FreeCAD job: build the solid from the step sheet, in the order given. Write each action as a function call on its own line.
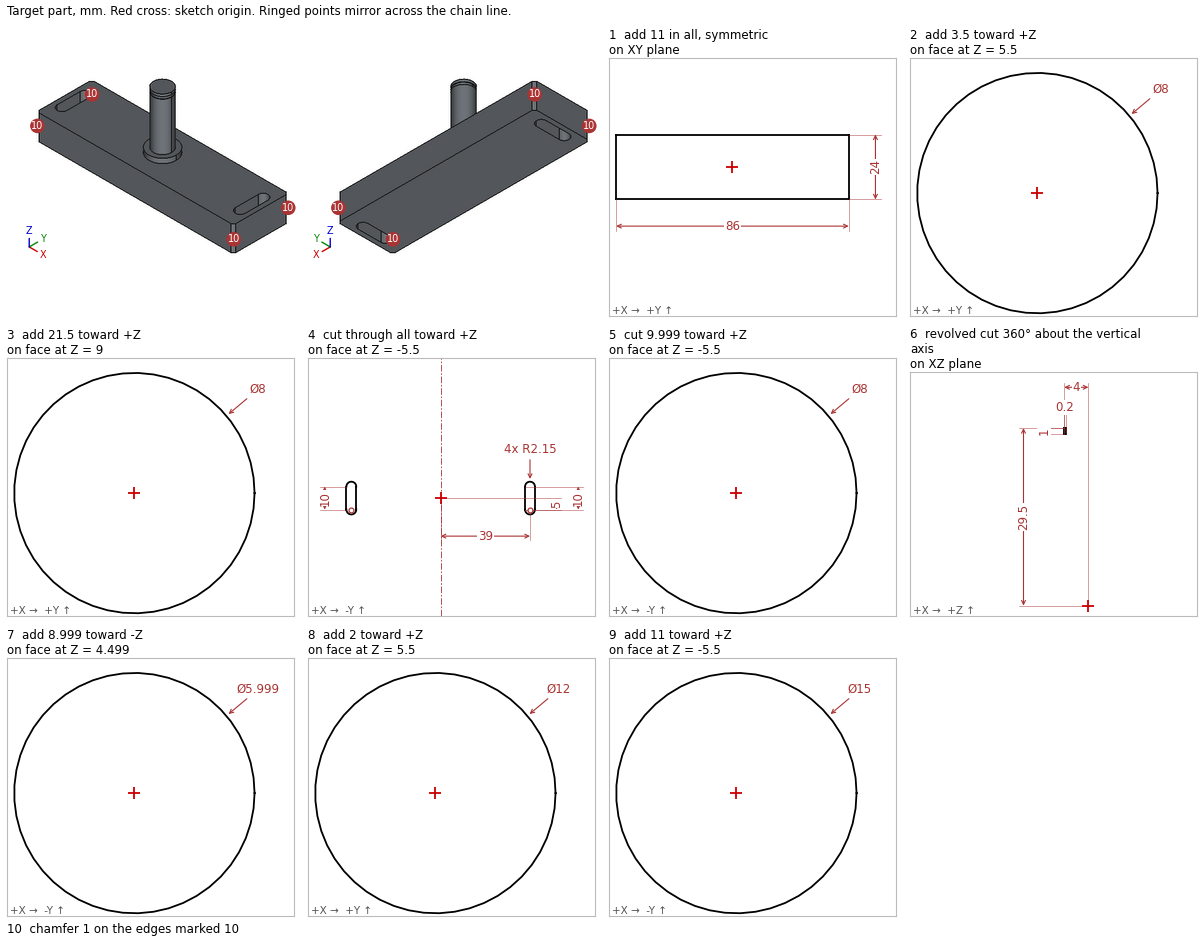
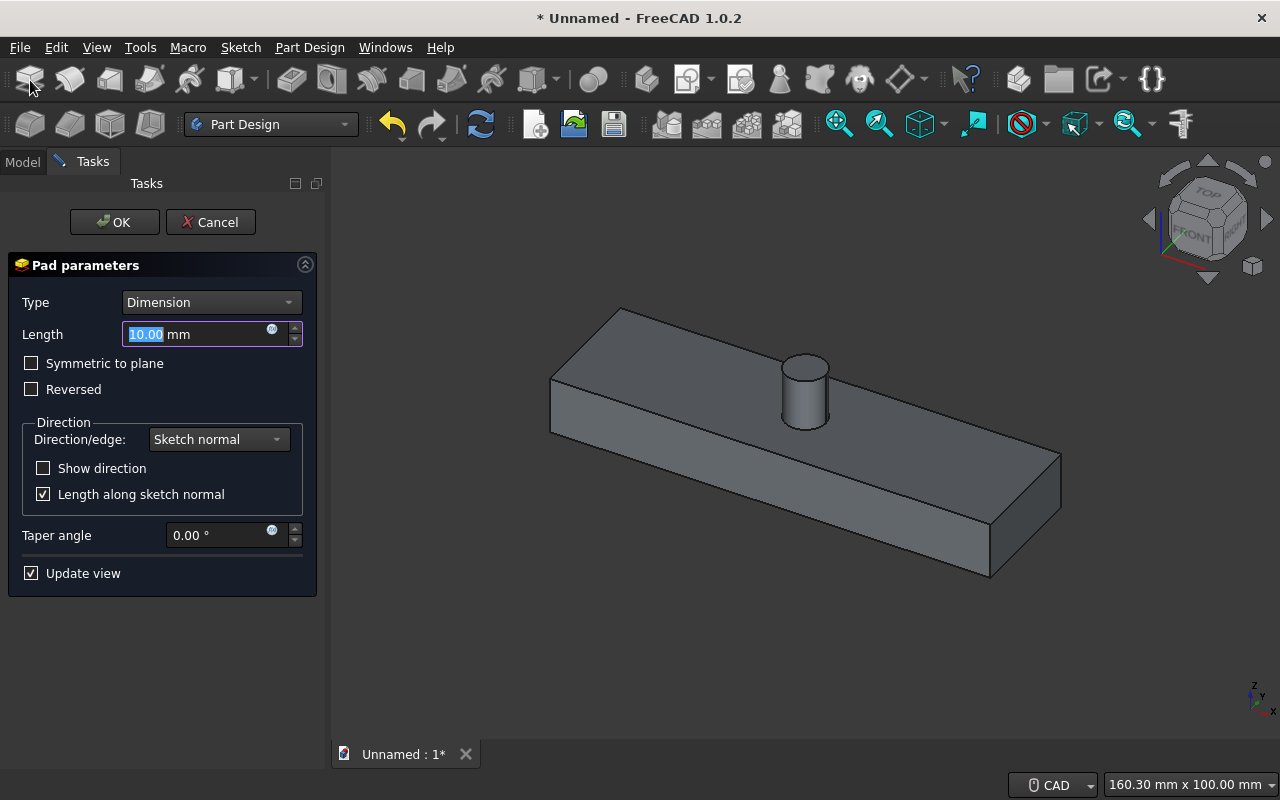
text(3.5)
key(Tab)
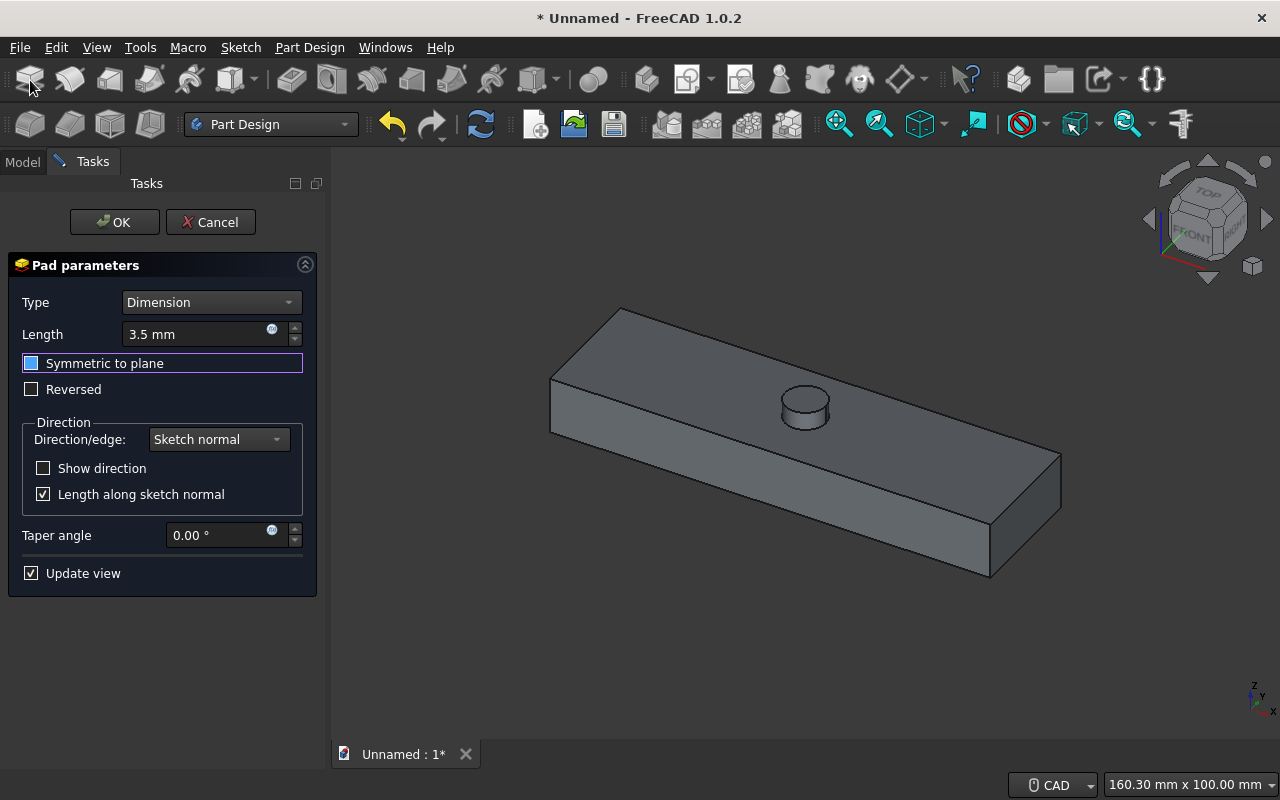
click(115, 222)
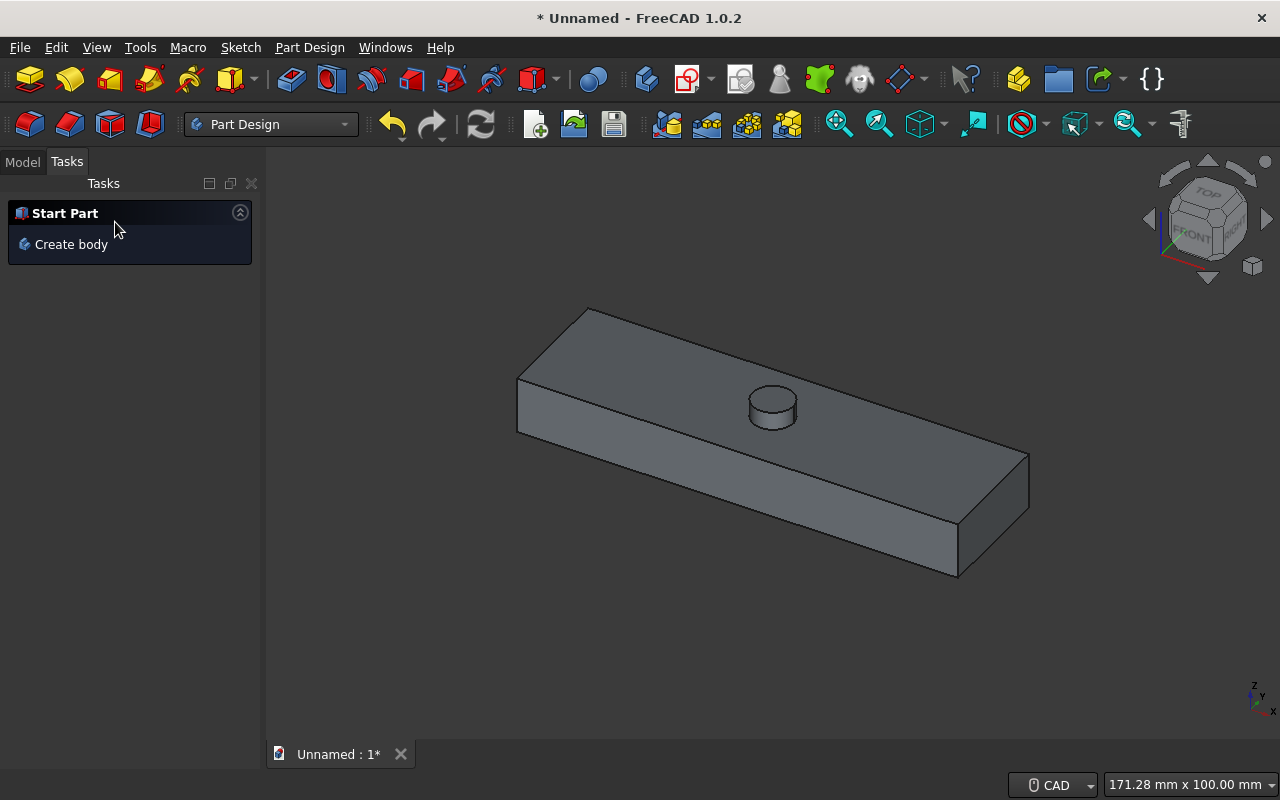
click(773, 398)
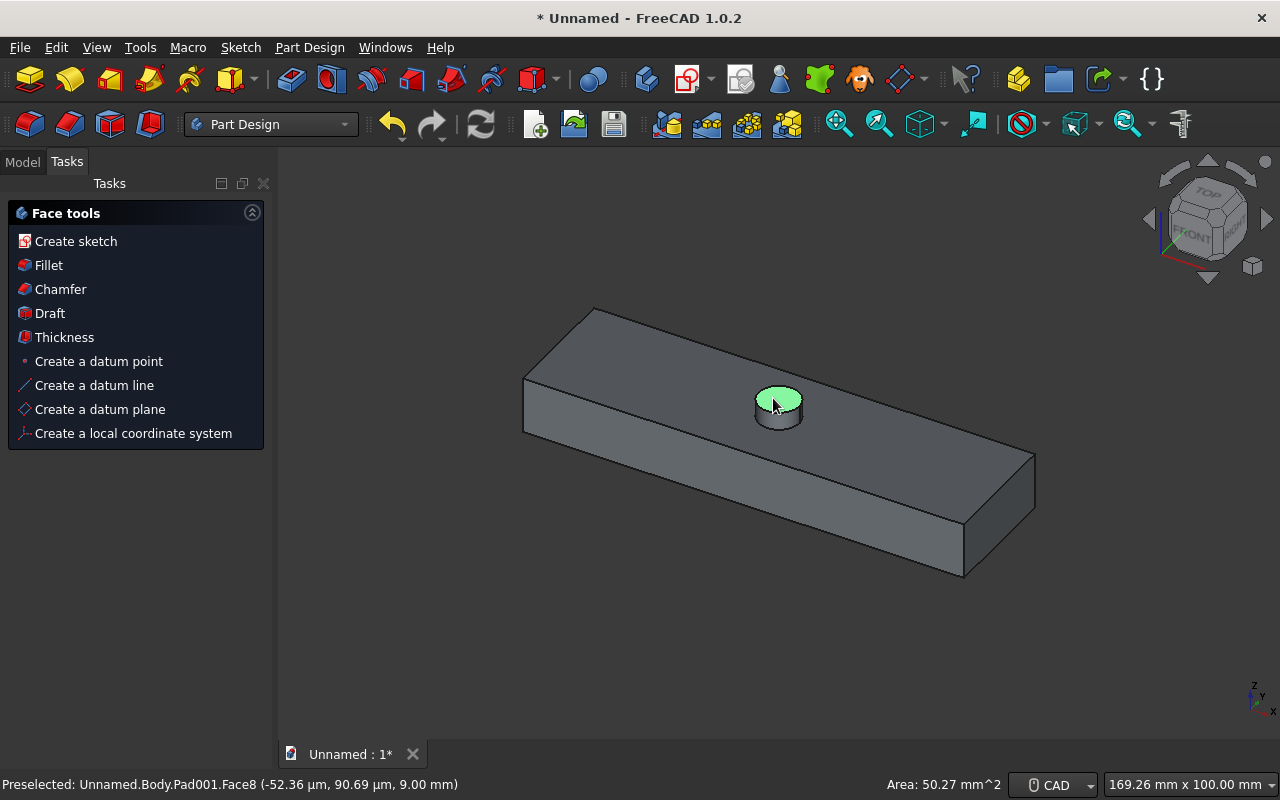
click(688, 80)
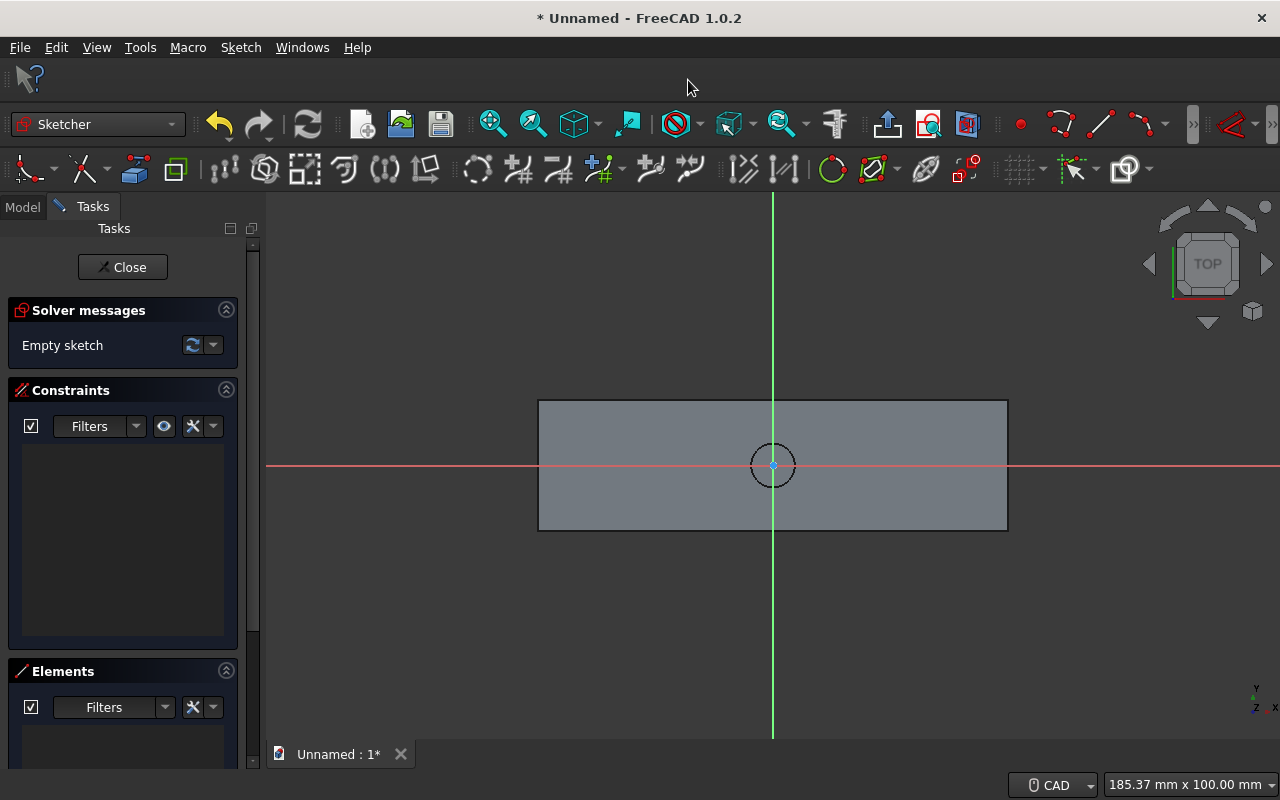
scroll(784, 466, up, 10)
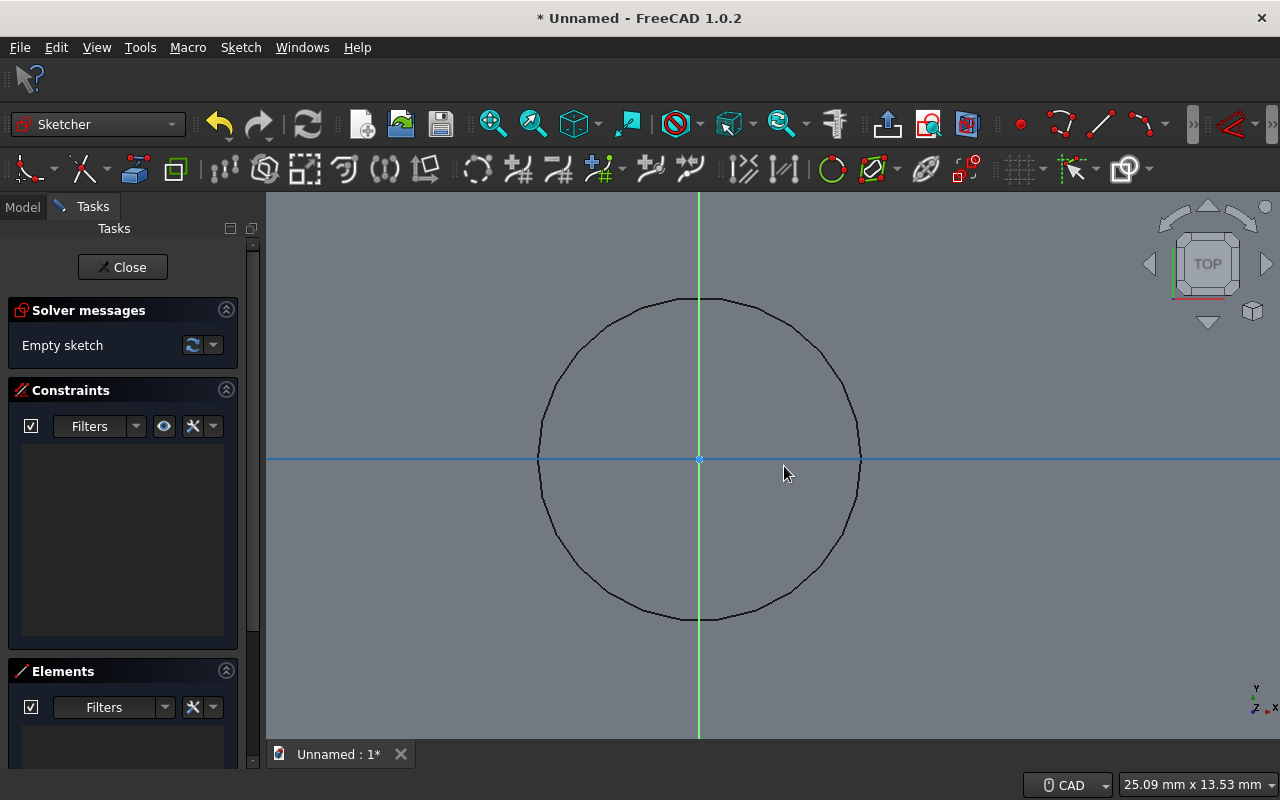
key(g)
key(c)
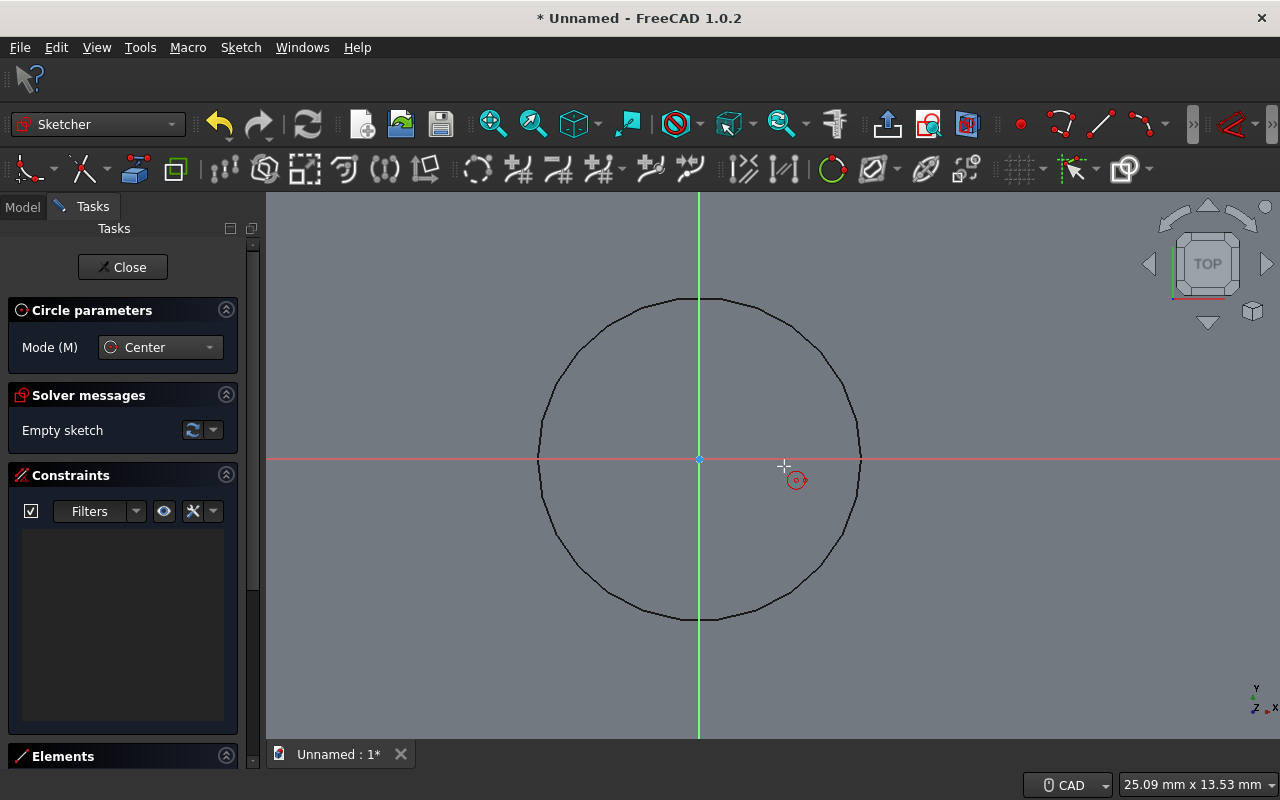
click(699, 459)
move(814, 345)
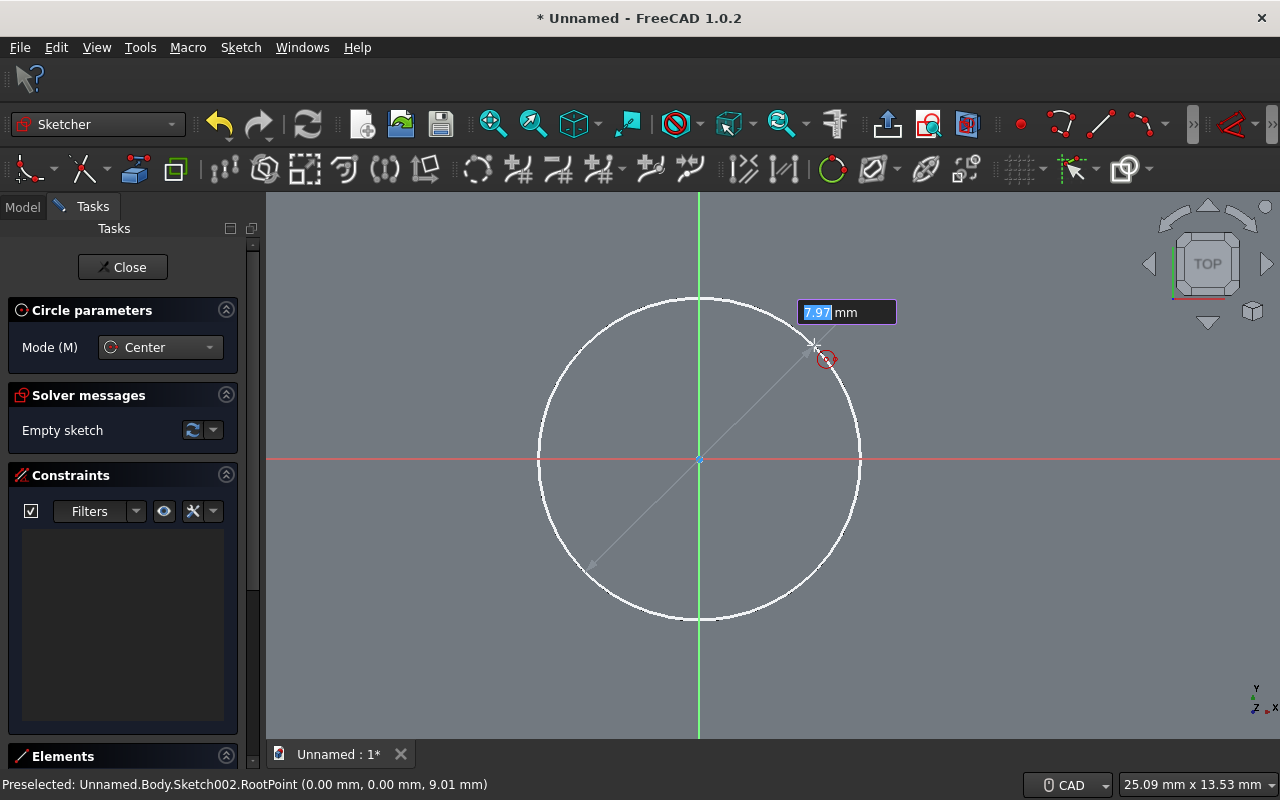
text(8)
key(Return)
key(Escape)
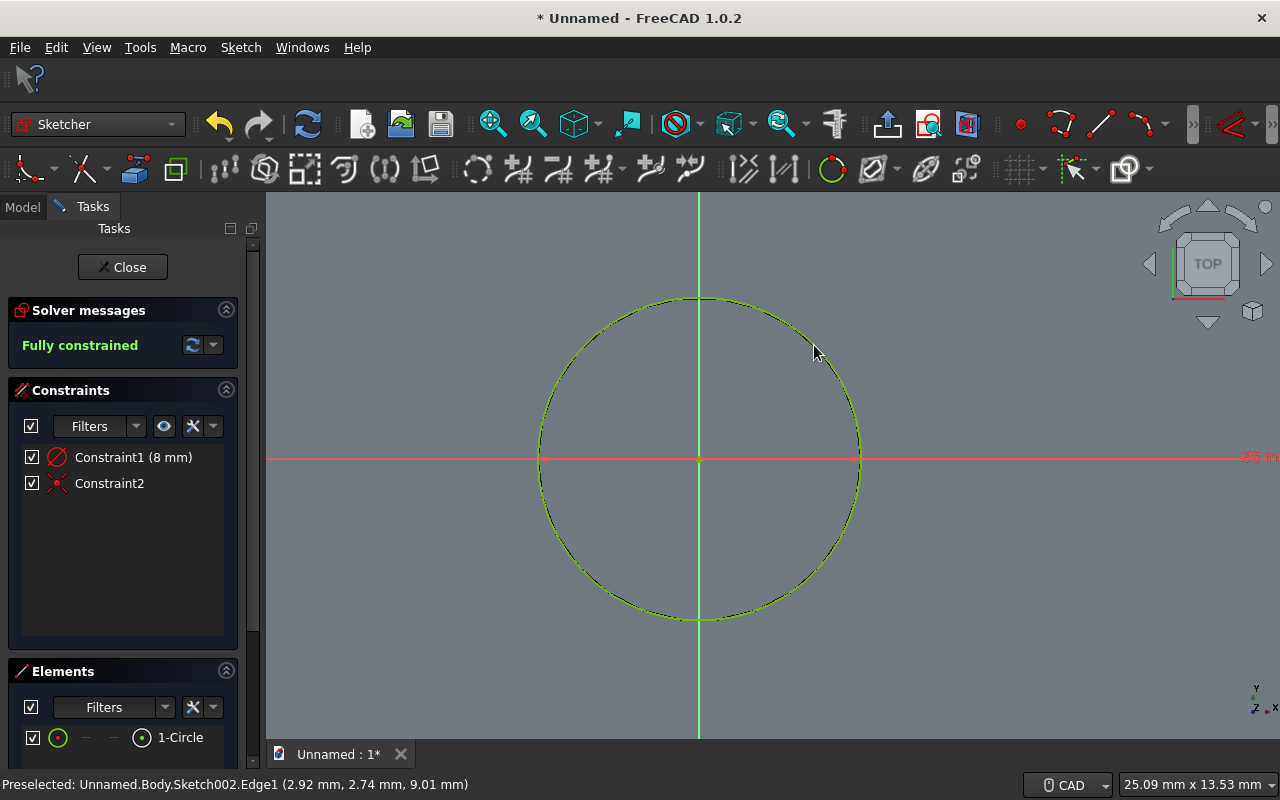
click(123, 267)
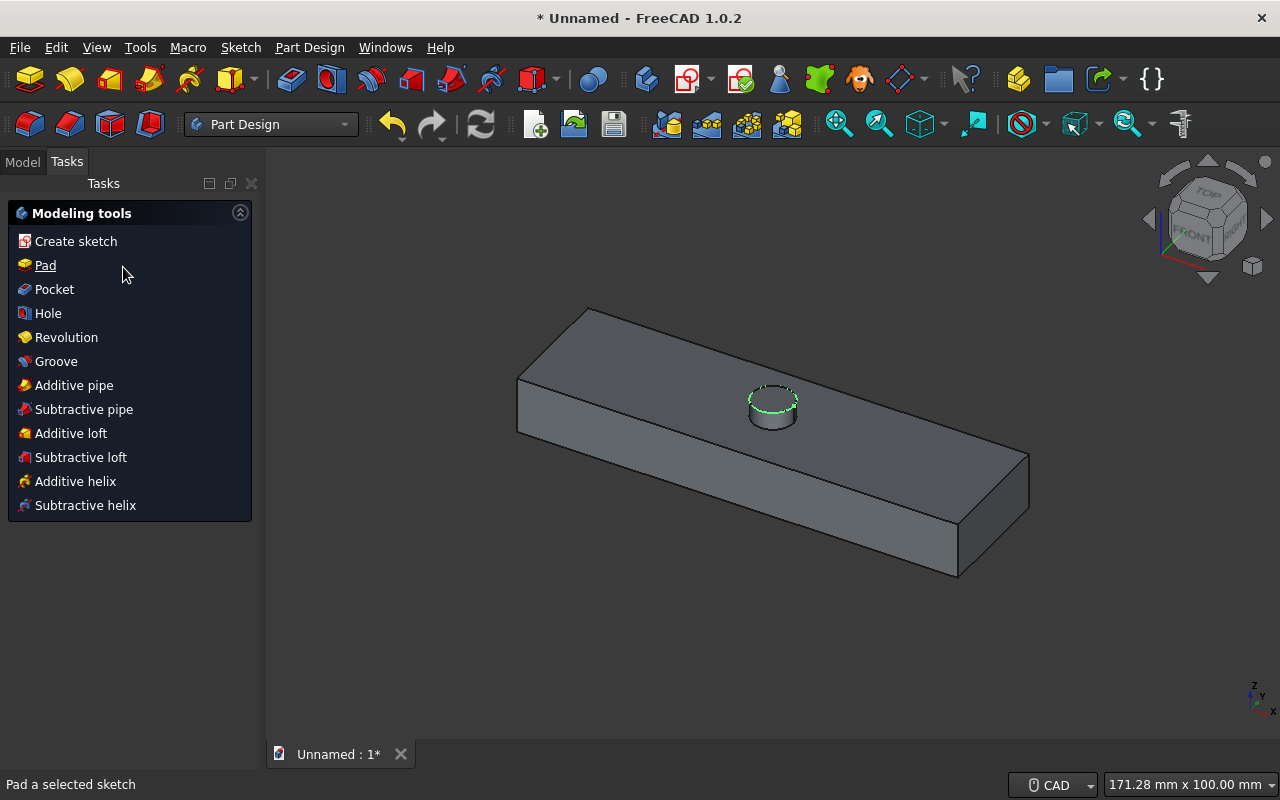
click(30, 80)